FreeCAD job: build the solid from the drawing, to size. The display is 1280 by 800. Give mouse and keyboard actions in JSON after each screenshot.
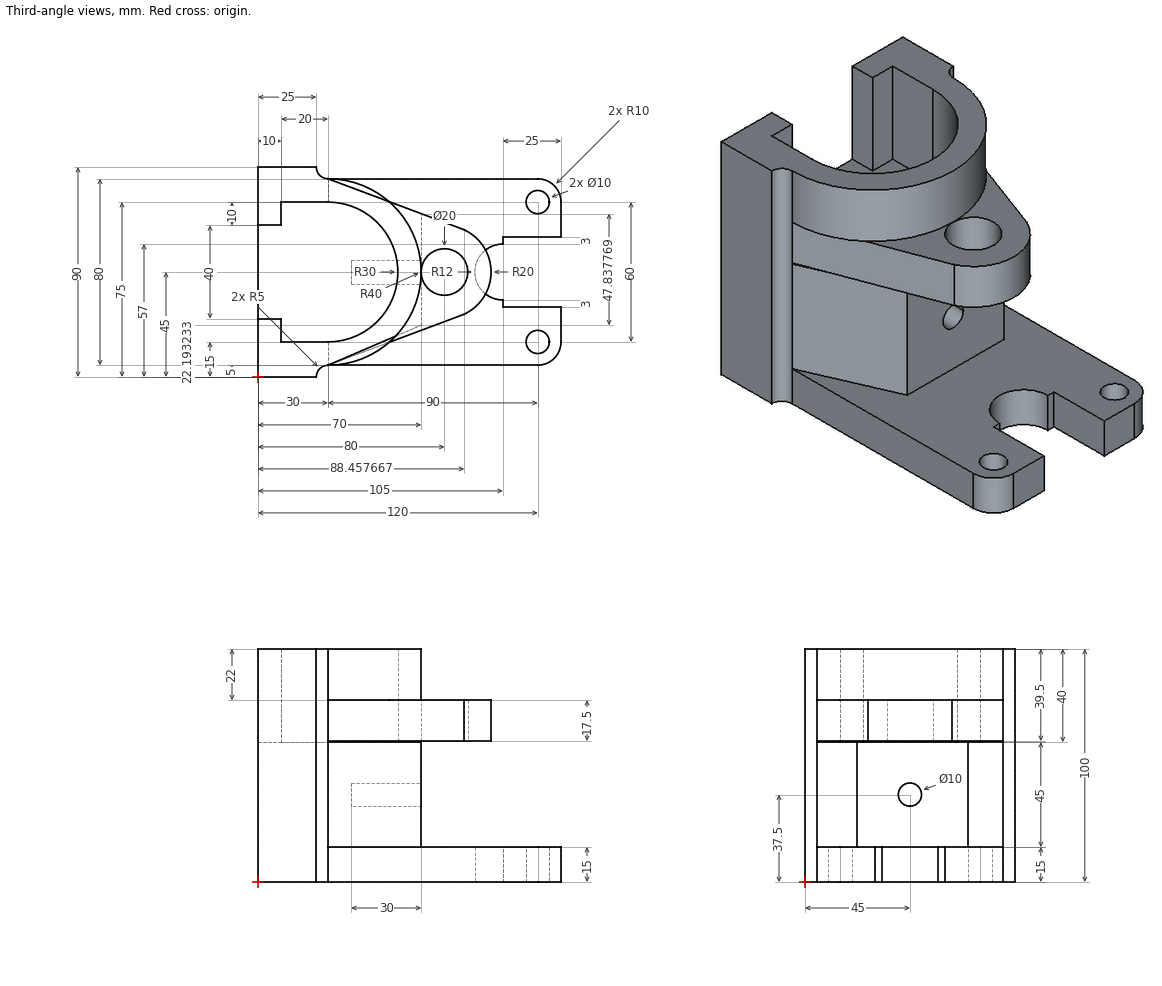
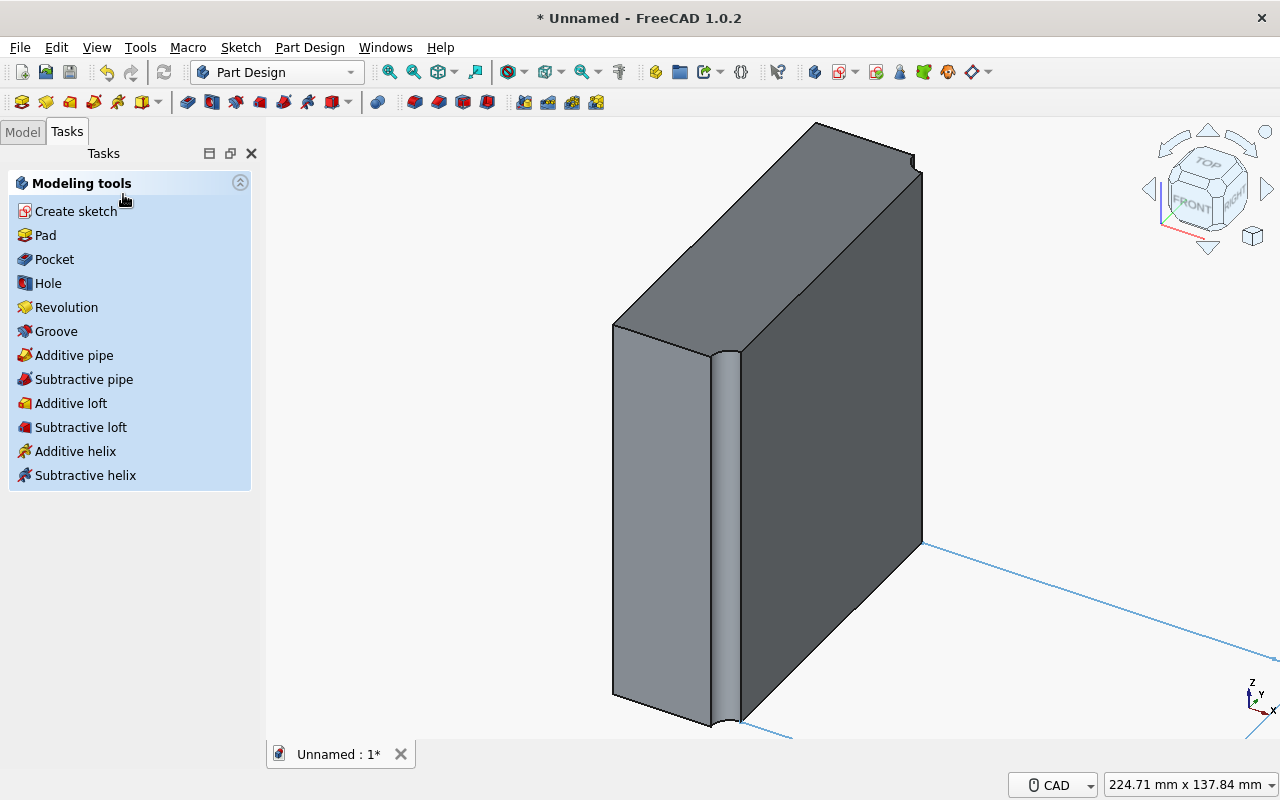
{"action": "left_click", "coordinate": [22, 102]}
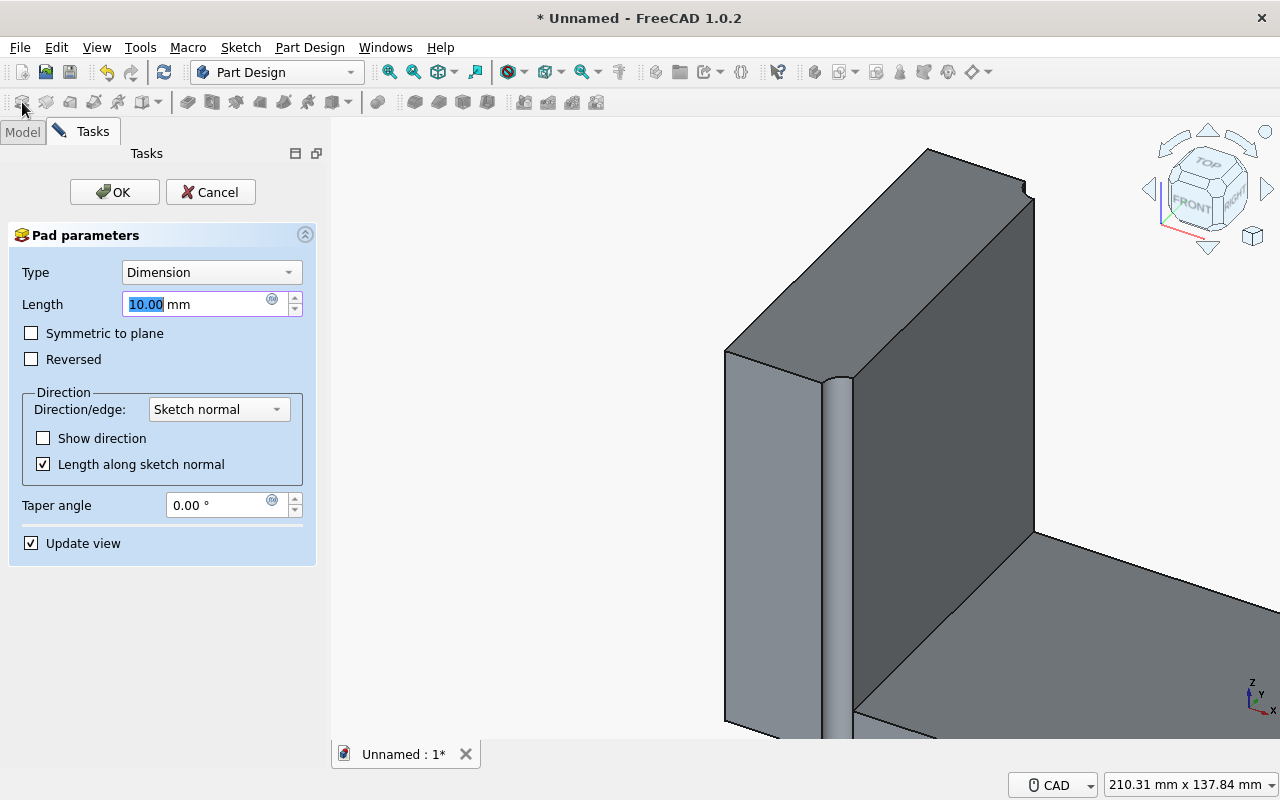
{"action": "type", "text": "15"}
{"action": "key", "text": "Tab"}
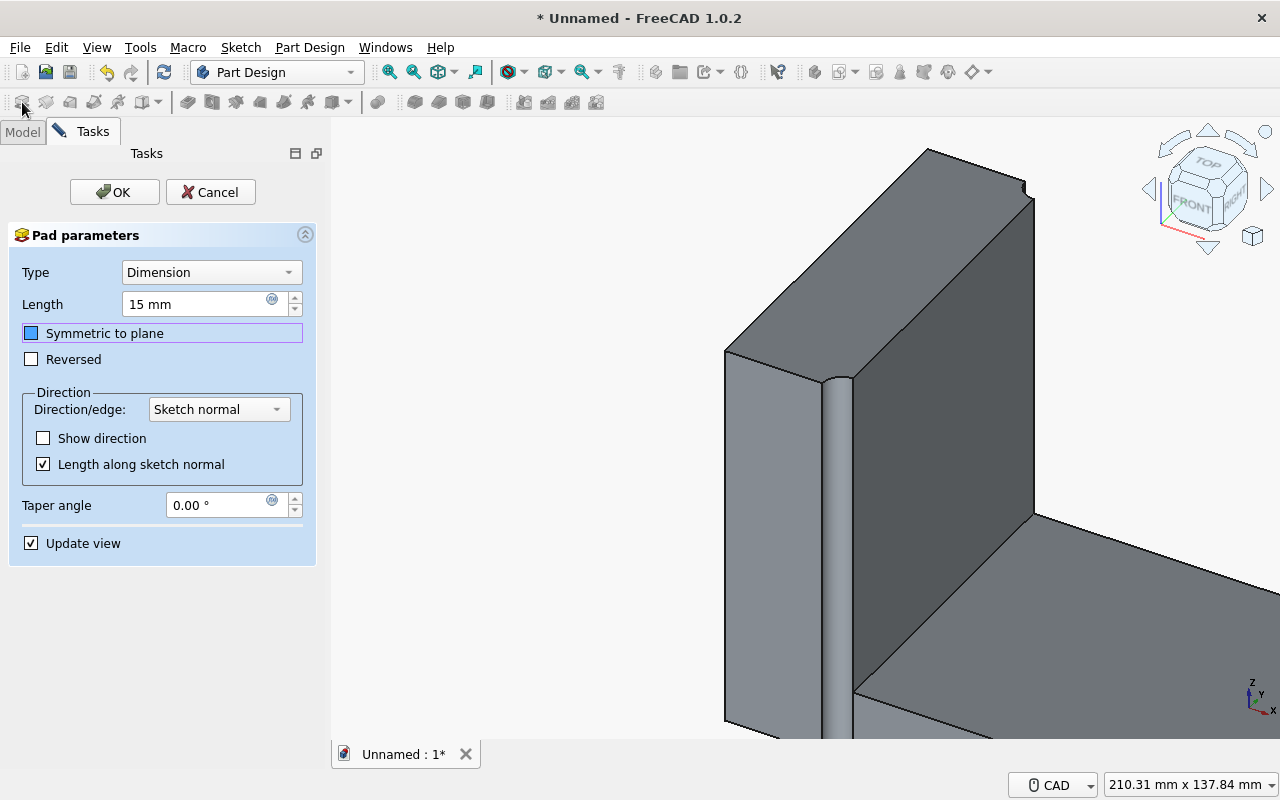
{"action": "left_click", "coordinate": [115, 192]}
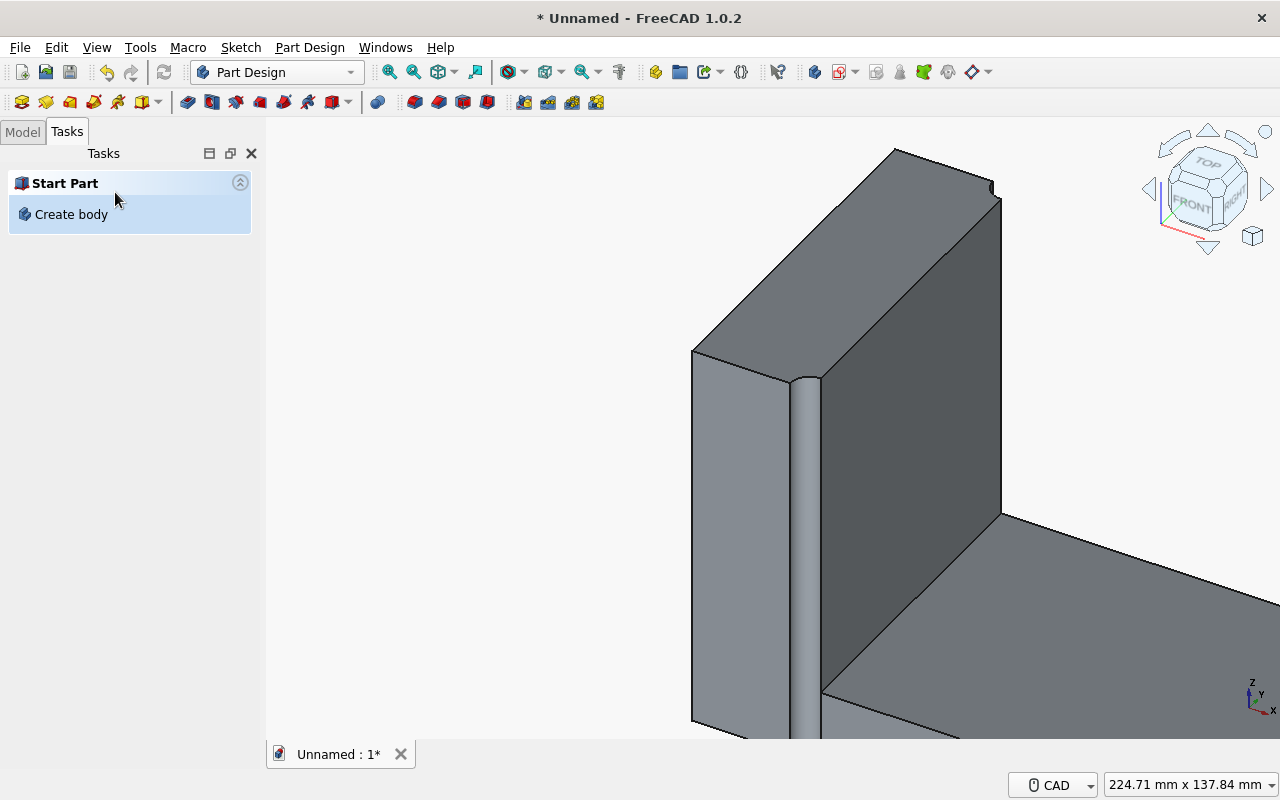
{"action": "left_click", "coordinate": [390, 72]}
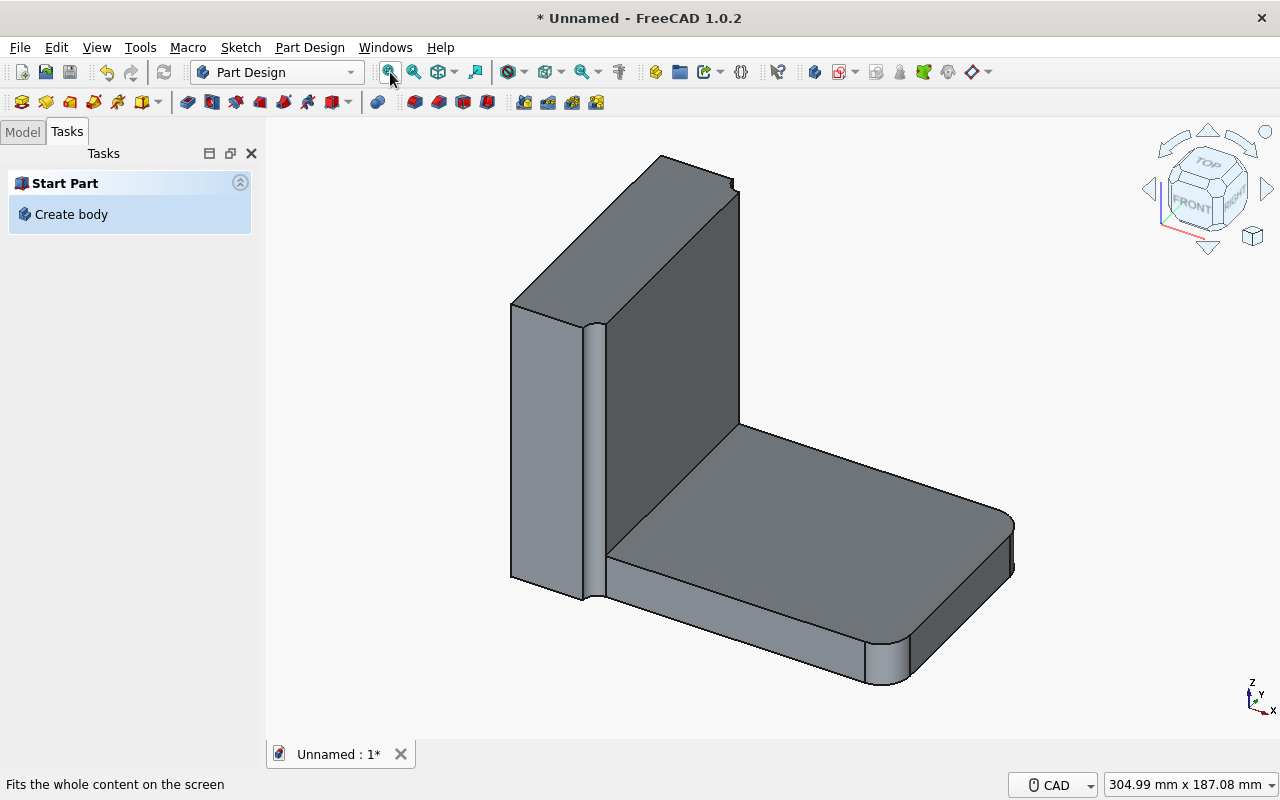
{"action": "left_click", "coordinate": [840, 72]}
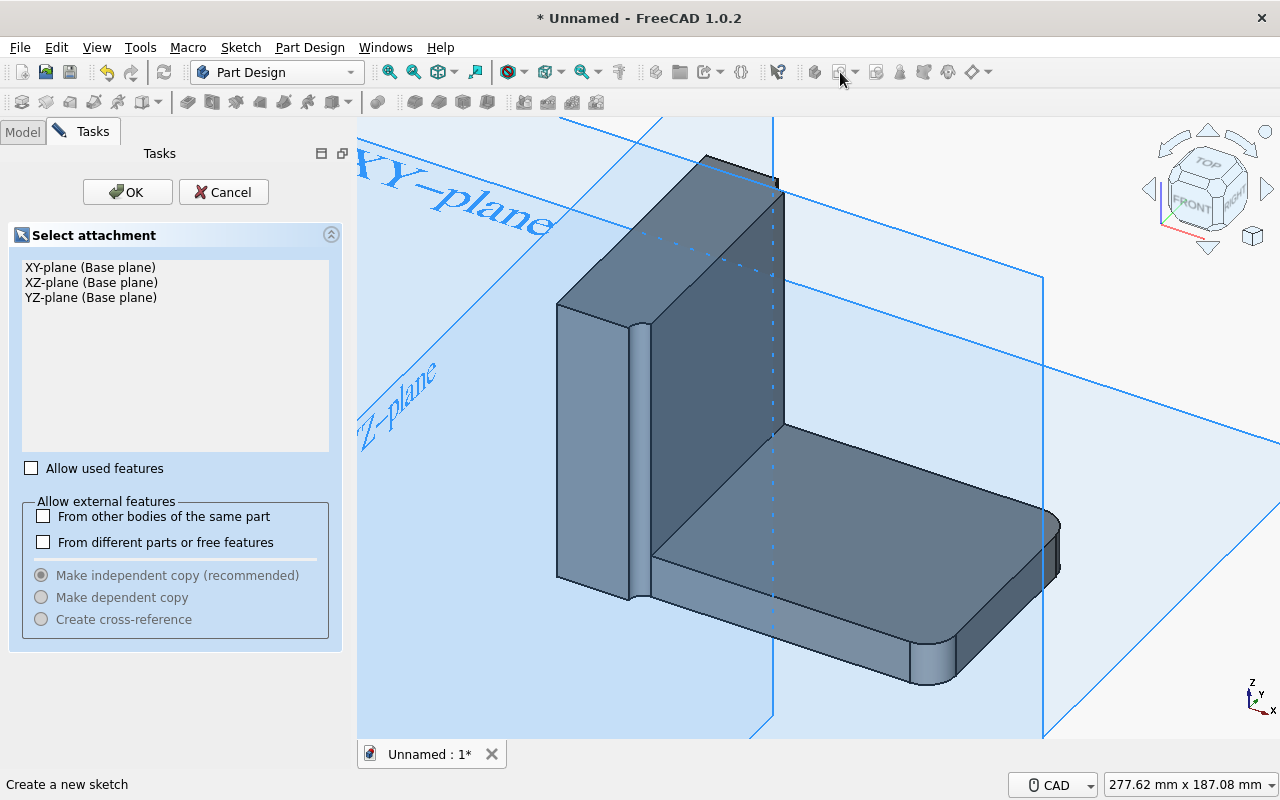
{"action": "left_click", "coordinate": [82, 268]}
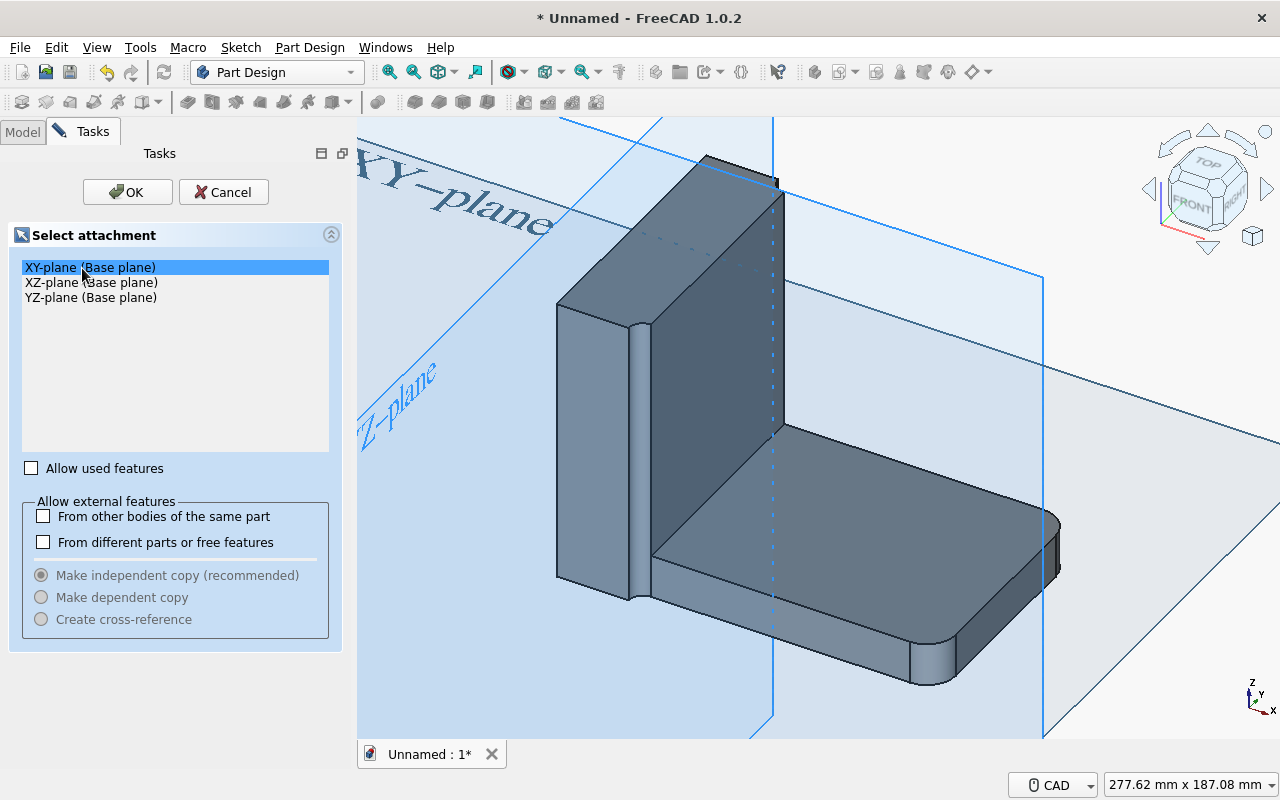
{"action": "left_click", "coordinate": [128, 192]}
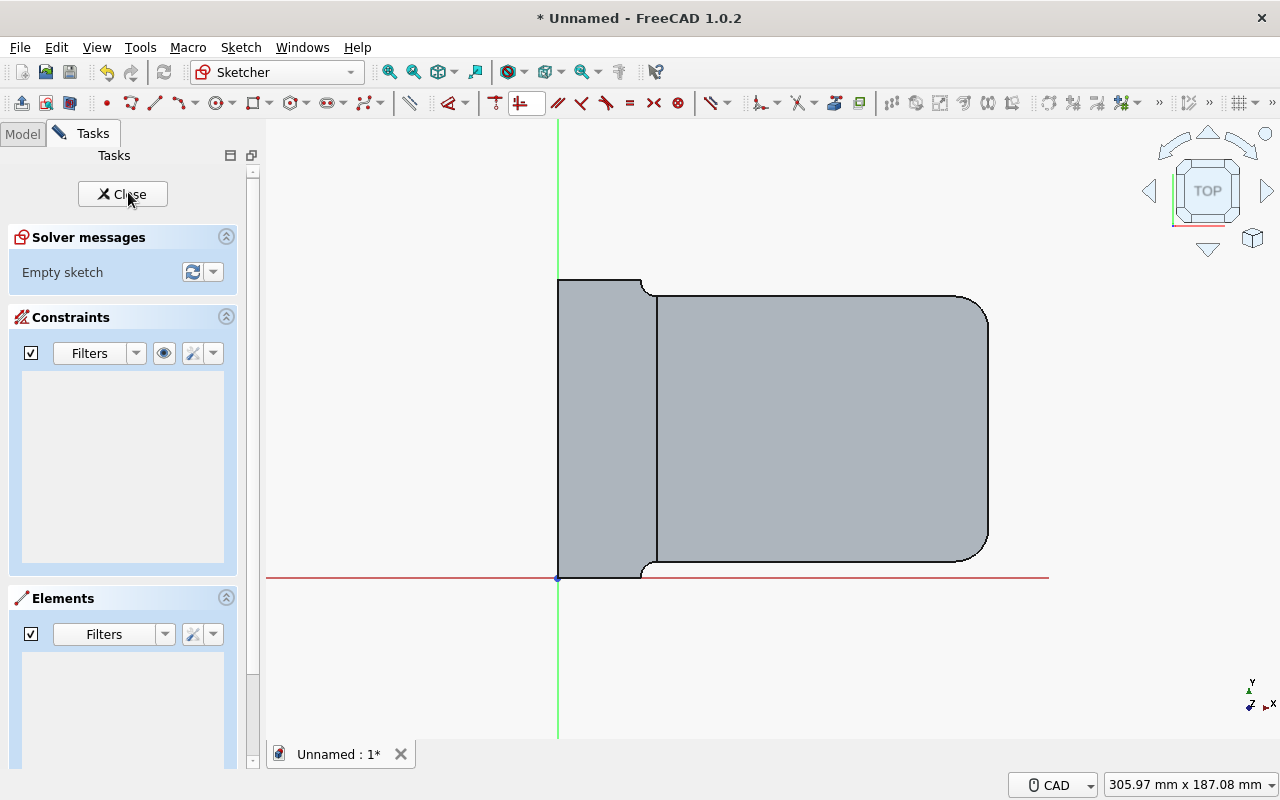
{"action": "left_click", "coordinate": [70, 104]}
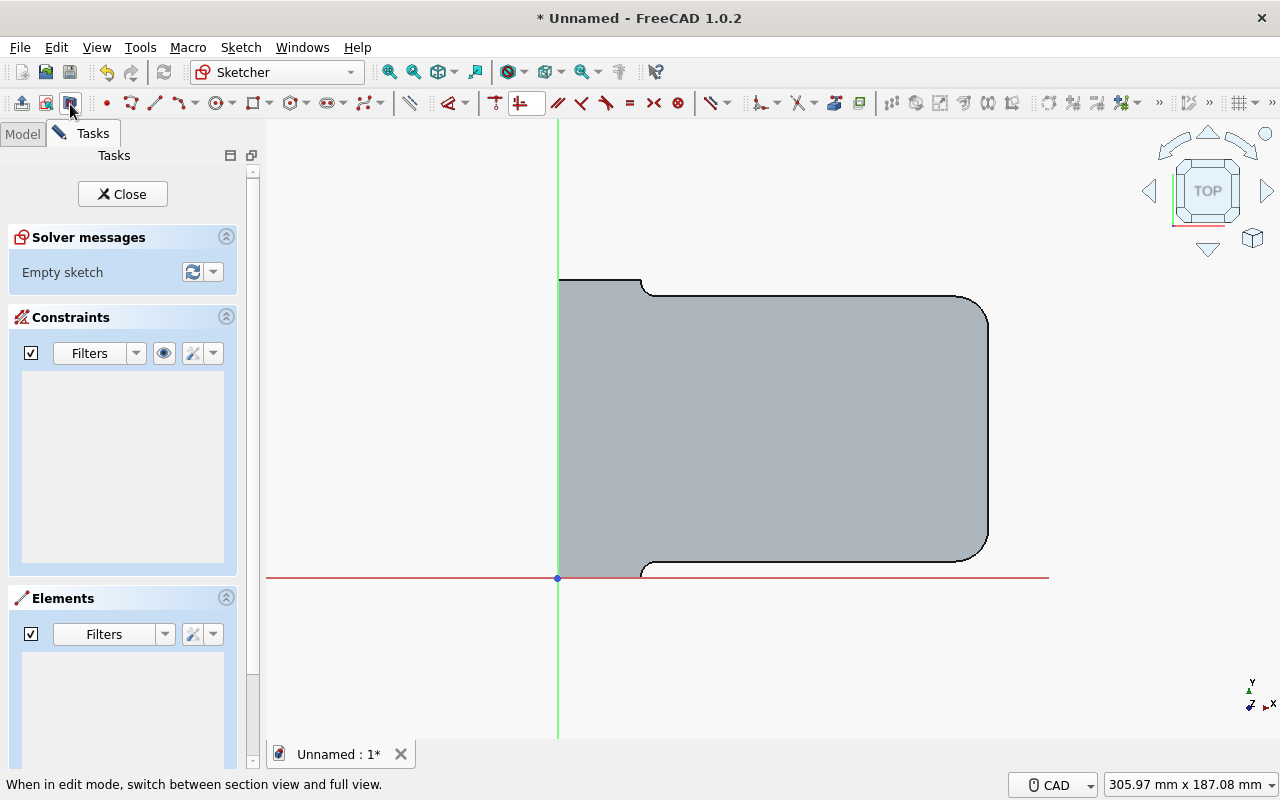
{"action": "scroll", "coordinate": [1000, 429], "scroll_direction": "up", "scroll_amount": 7}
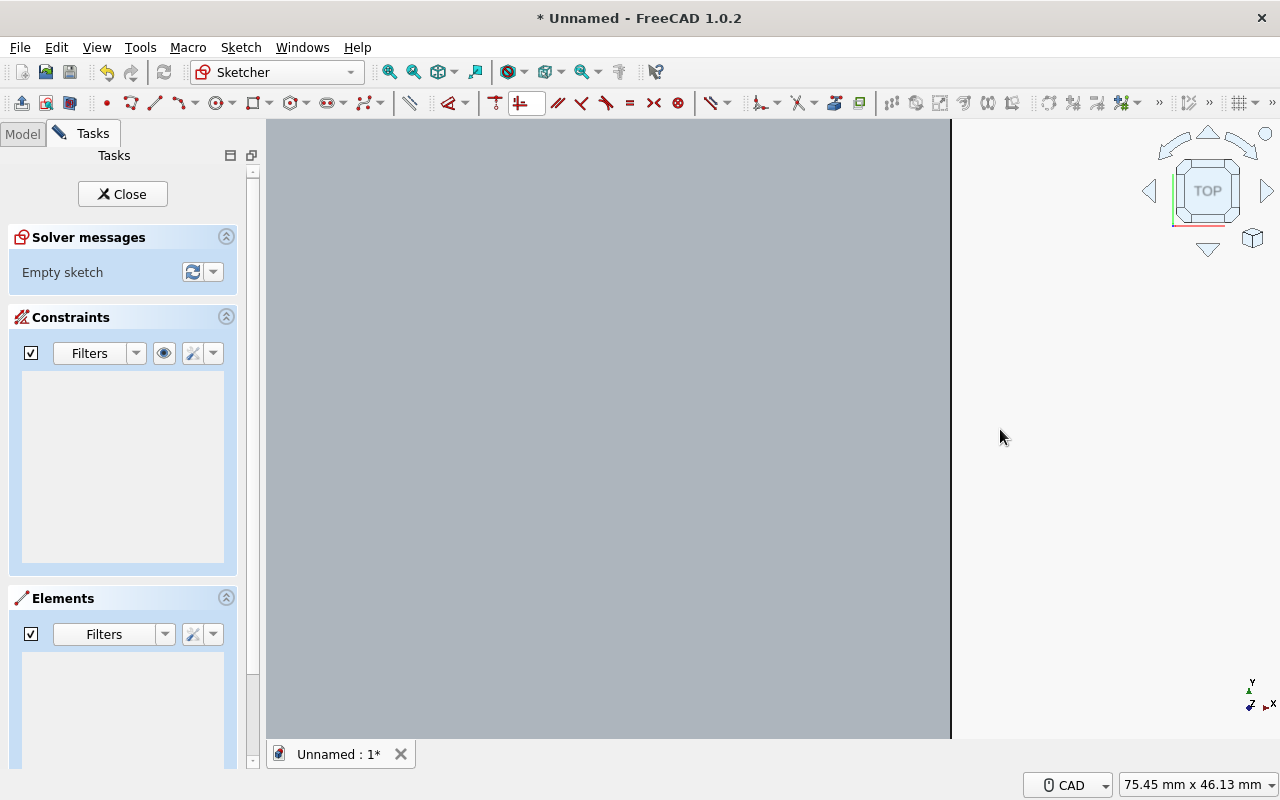
{"action": "key", "text": "g m"}